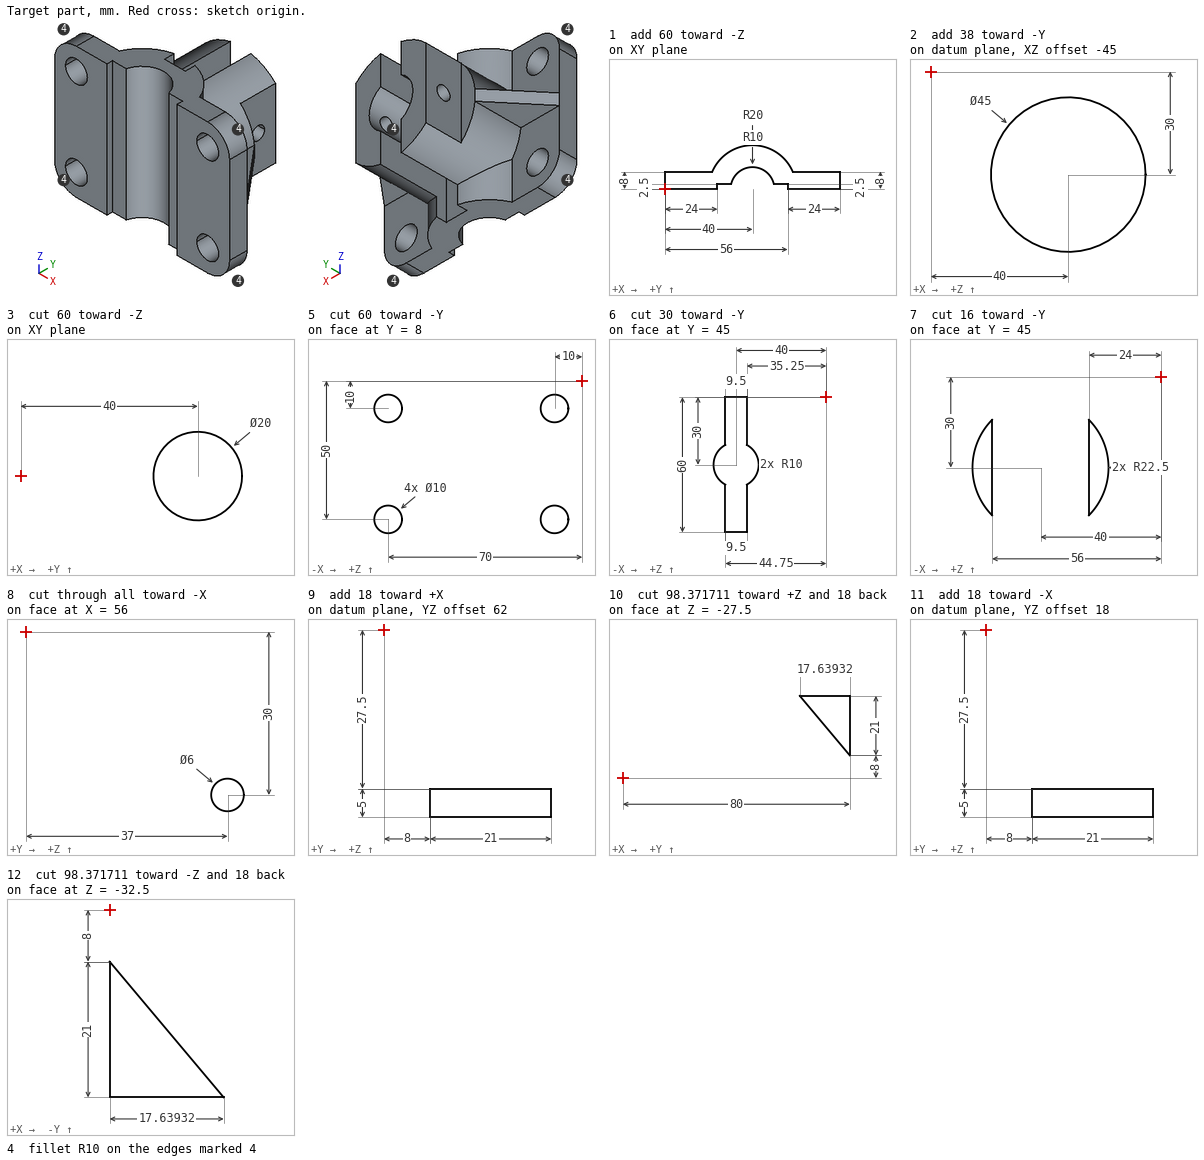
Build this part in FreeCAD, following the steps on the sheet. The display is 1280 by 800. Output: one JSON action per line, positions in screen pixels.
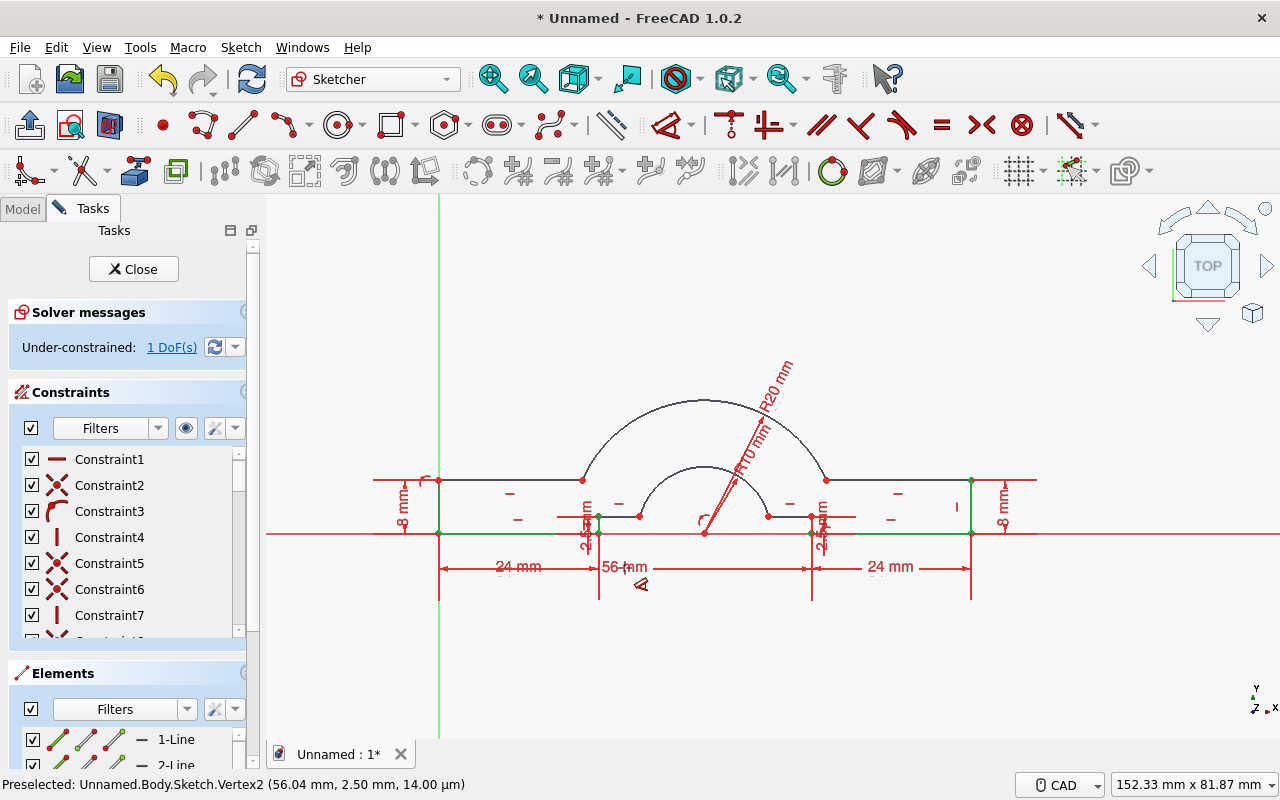
{"action": "left_click", "coordinate": [704, 534]}
{"action": "left_click", "coordinate": [572, 500]}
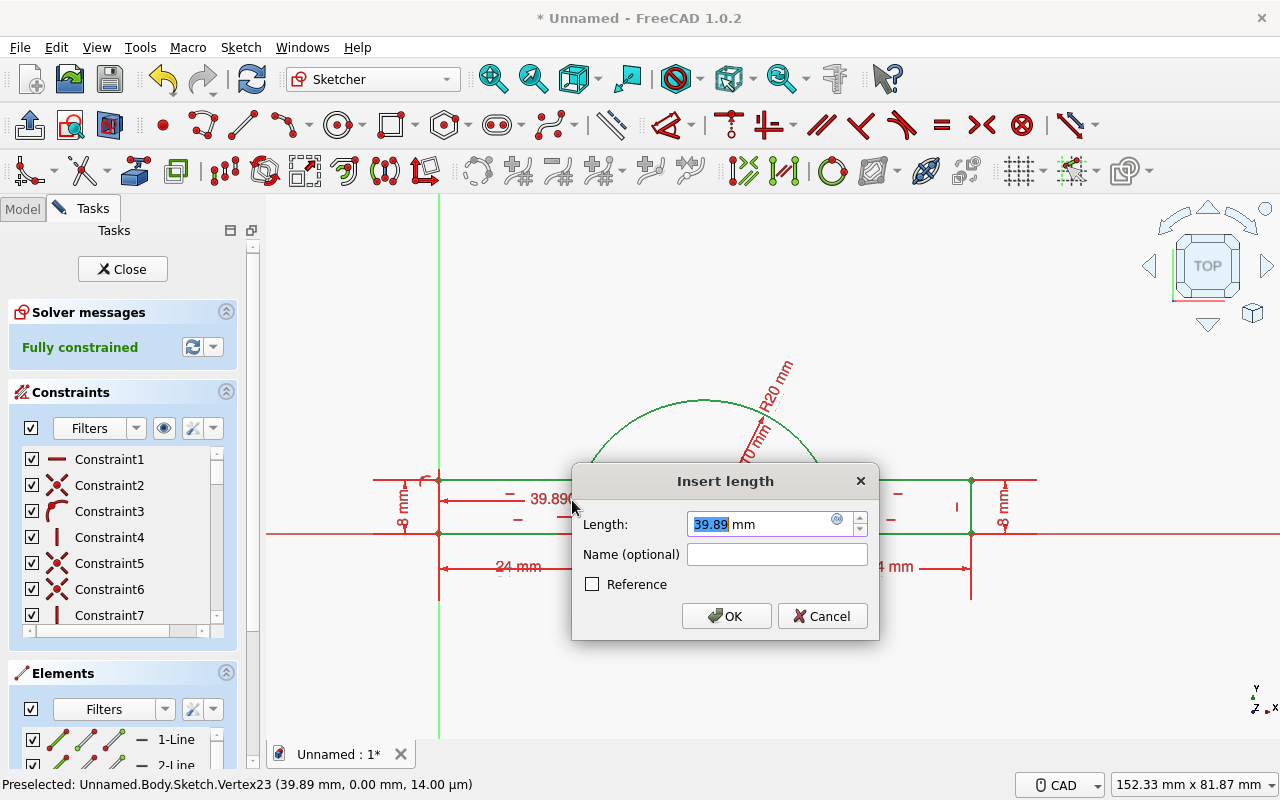
{"action": "type", "text": "40"}
{"action": "key", "text": "Return"}
{"action": "key", "text": "Escape"}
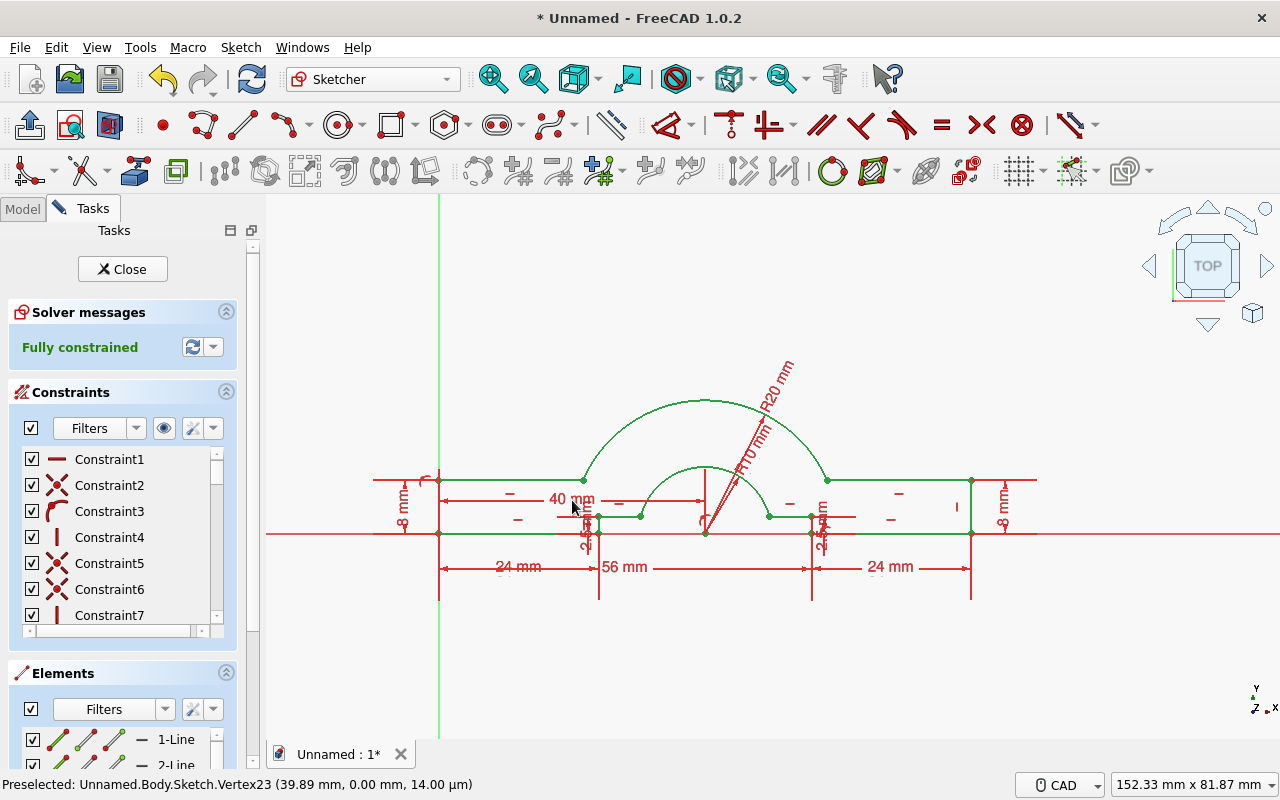
{"action": "left_click", "coordinate": [123, 269]}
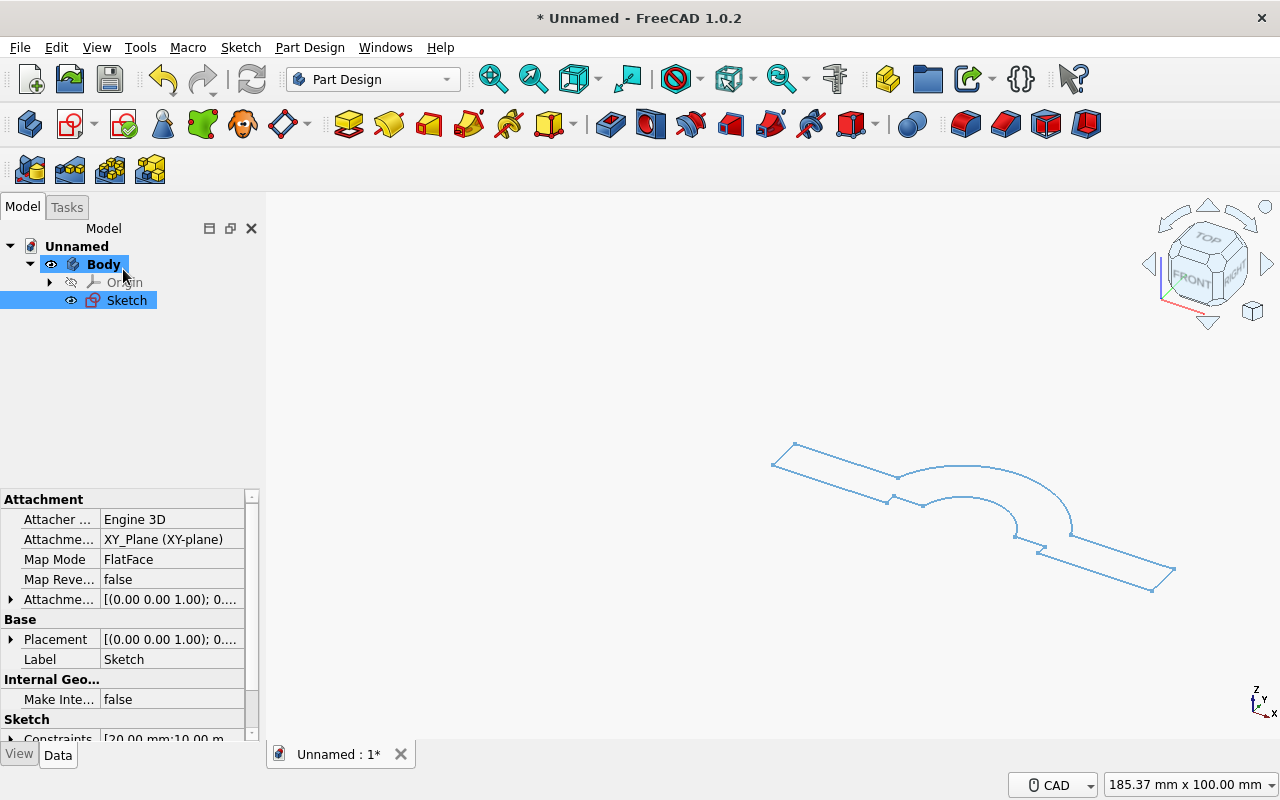
{"action": "left_click", "coordinate": [350, 124]}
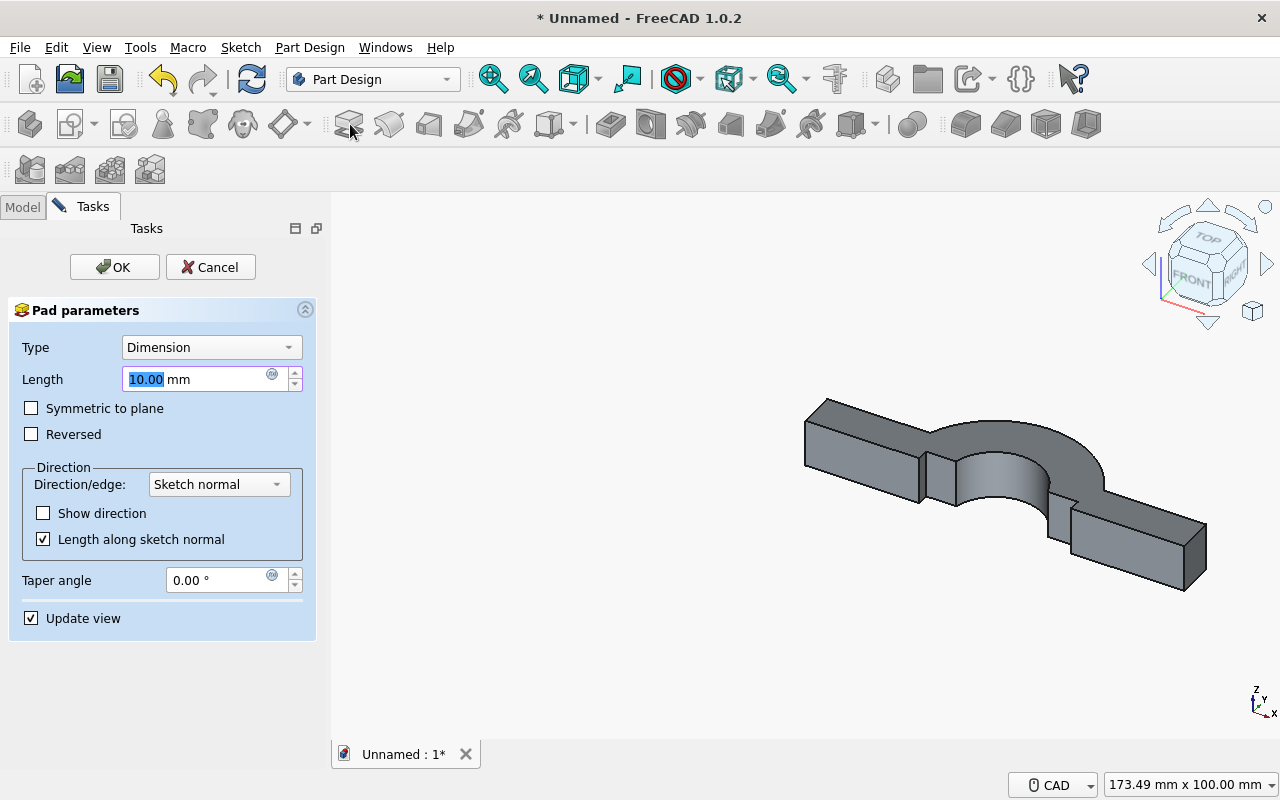
{"action": "type", "text": "60"}
{"action": "key", "text": "Tab"}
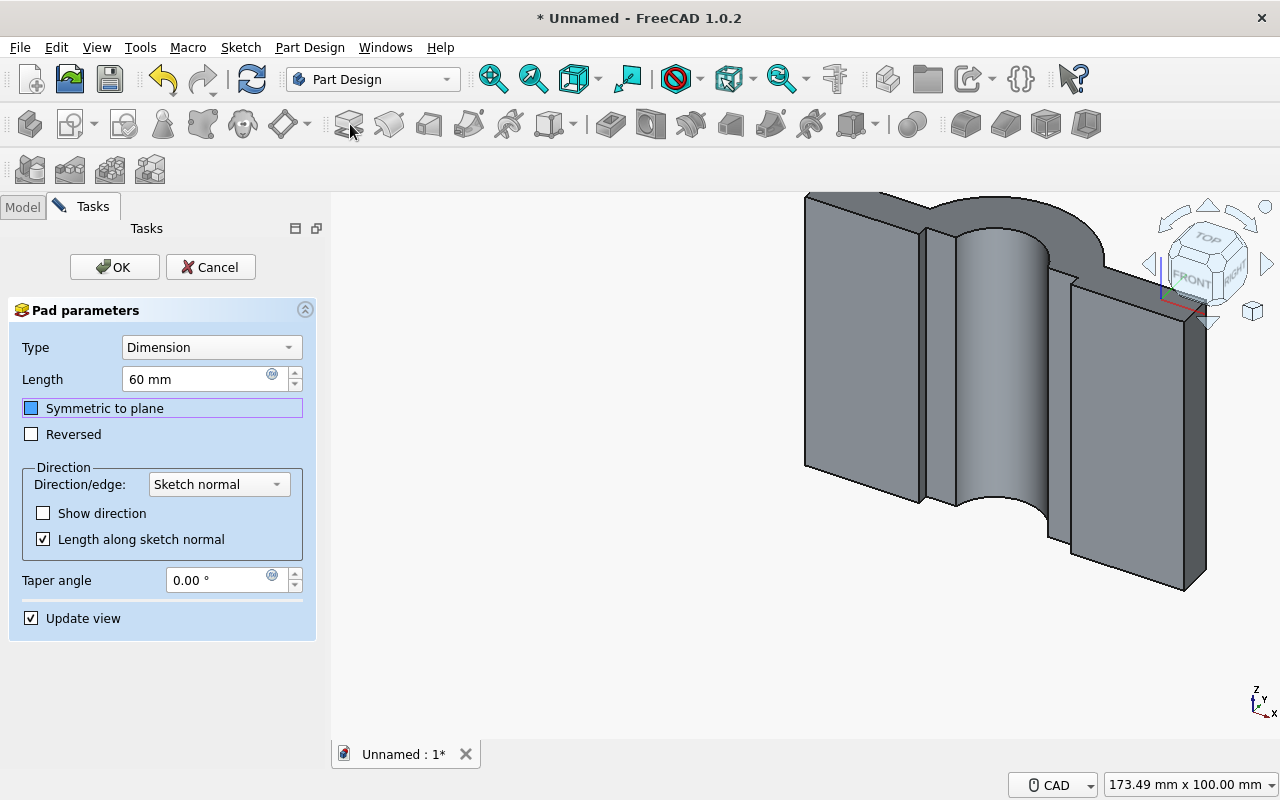
{"action": "left_click", "coordinate": [30, 434]}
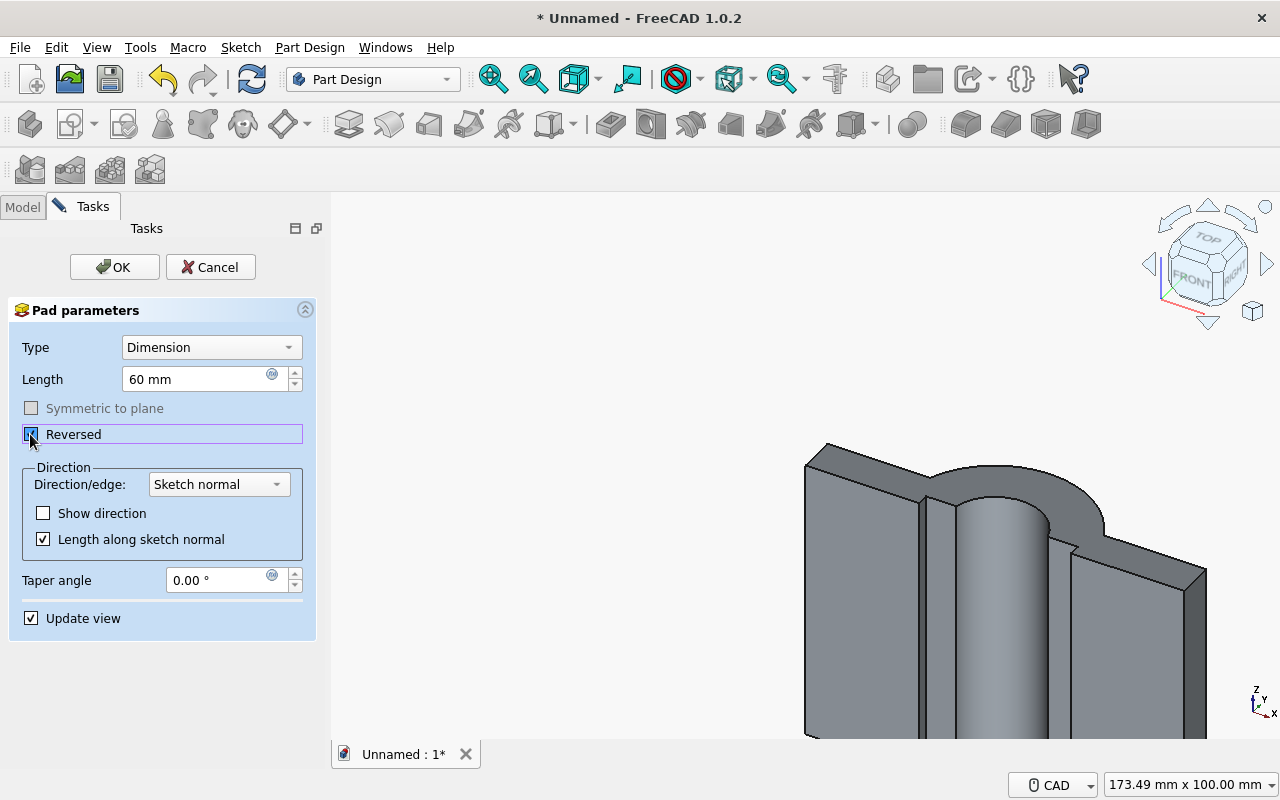
{"action": "left_click", "coordinate": [115, 267]}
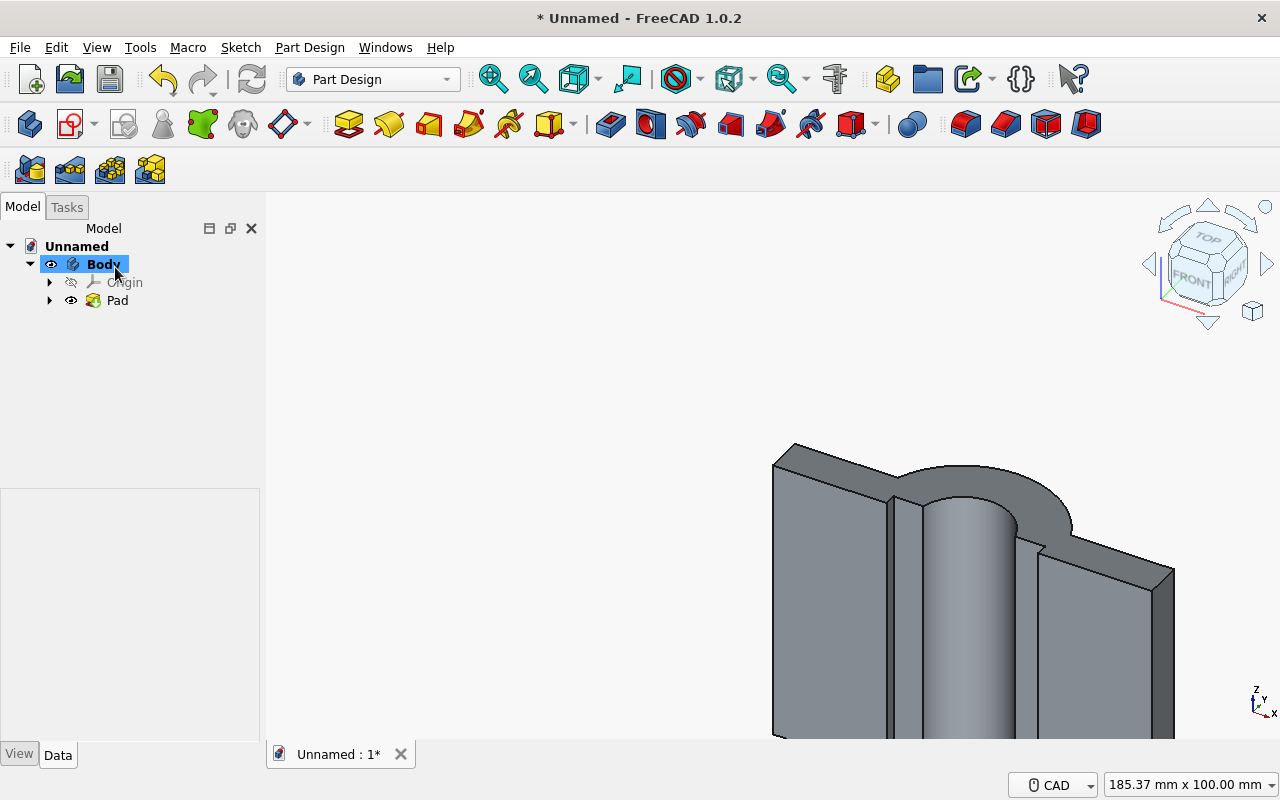
{"action": "left_click", "coordinate": [494, 80]}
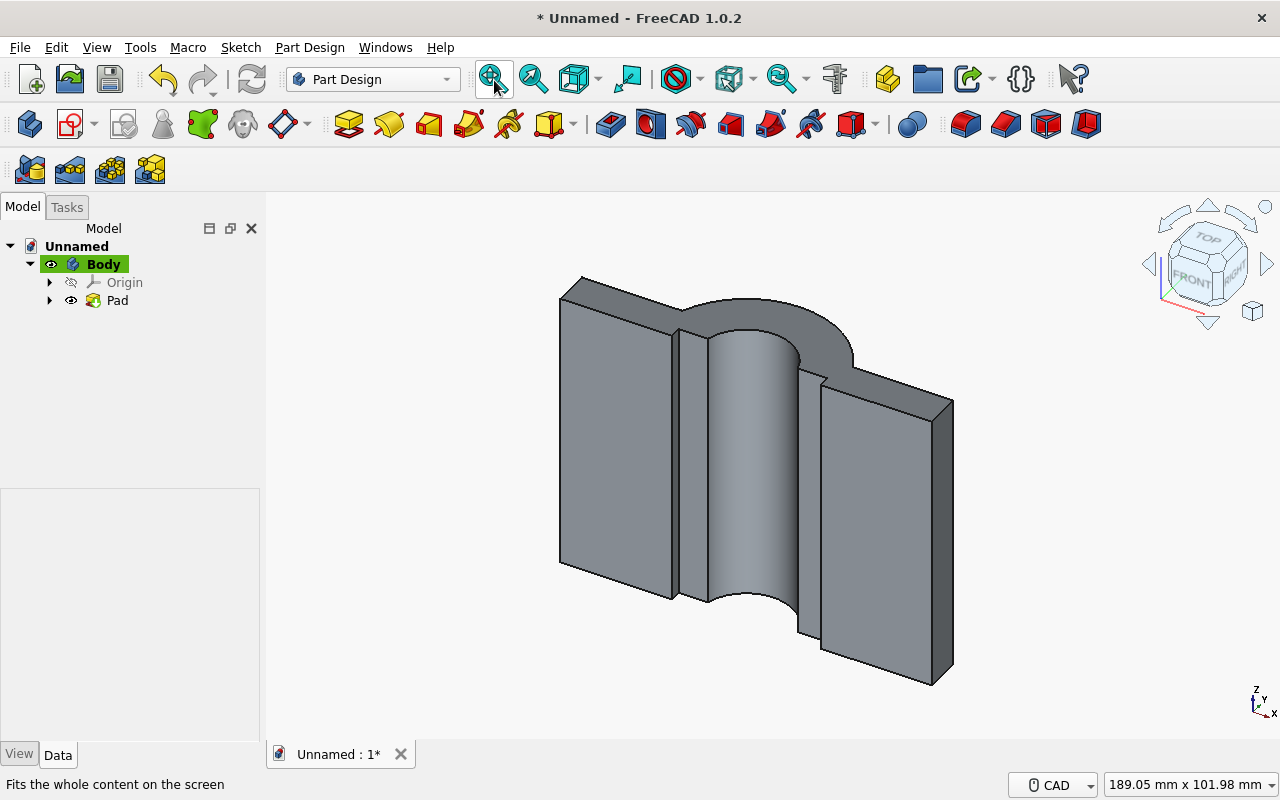
{"action": "left_click", "coordinate": [50, 282]}